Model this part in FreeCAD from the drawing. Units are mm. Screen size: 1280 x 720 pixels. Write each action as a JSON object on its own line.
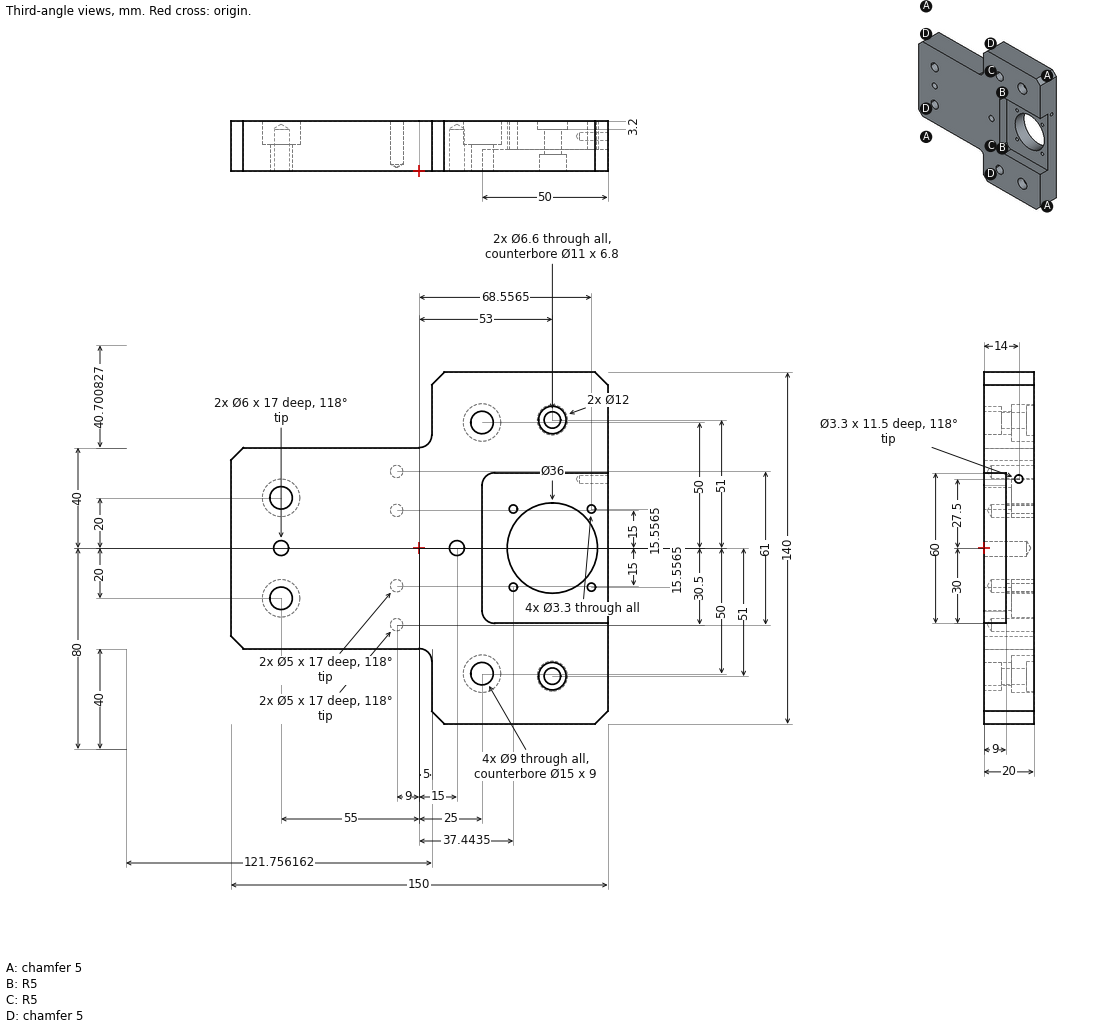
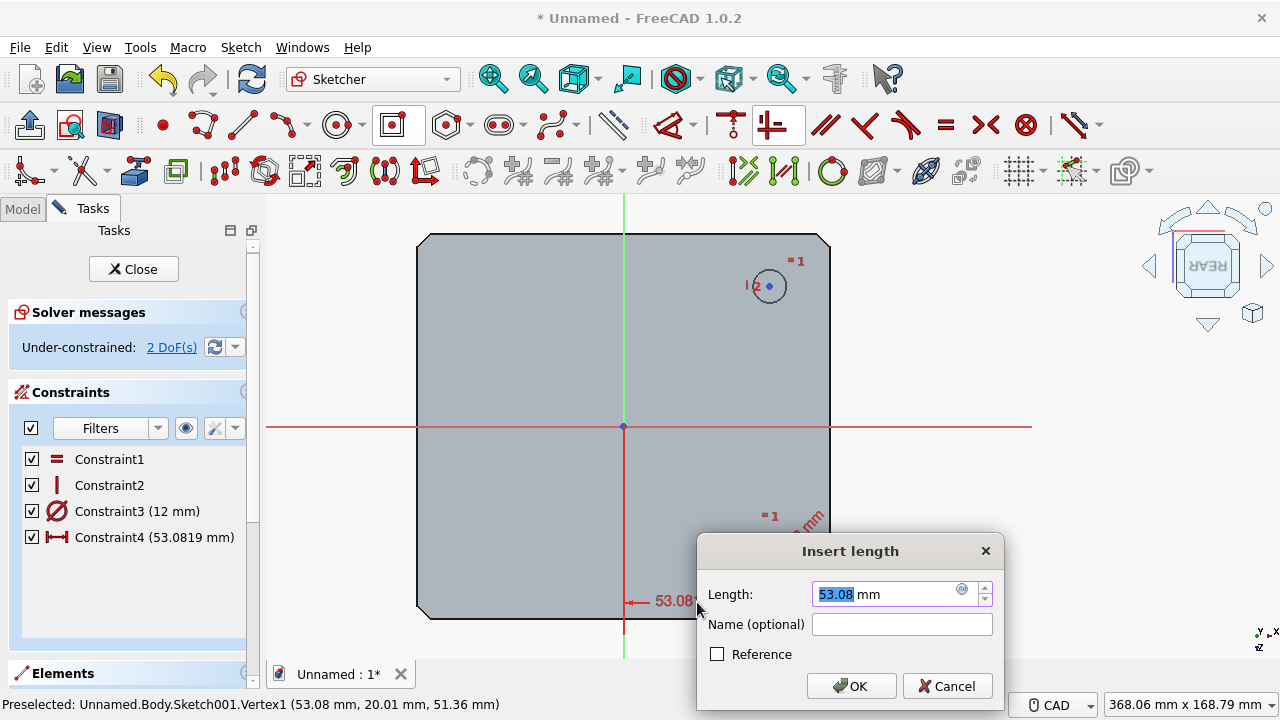
{"action": "type", "text": "53"}
{"action": "key", "text": "Return"}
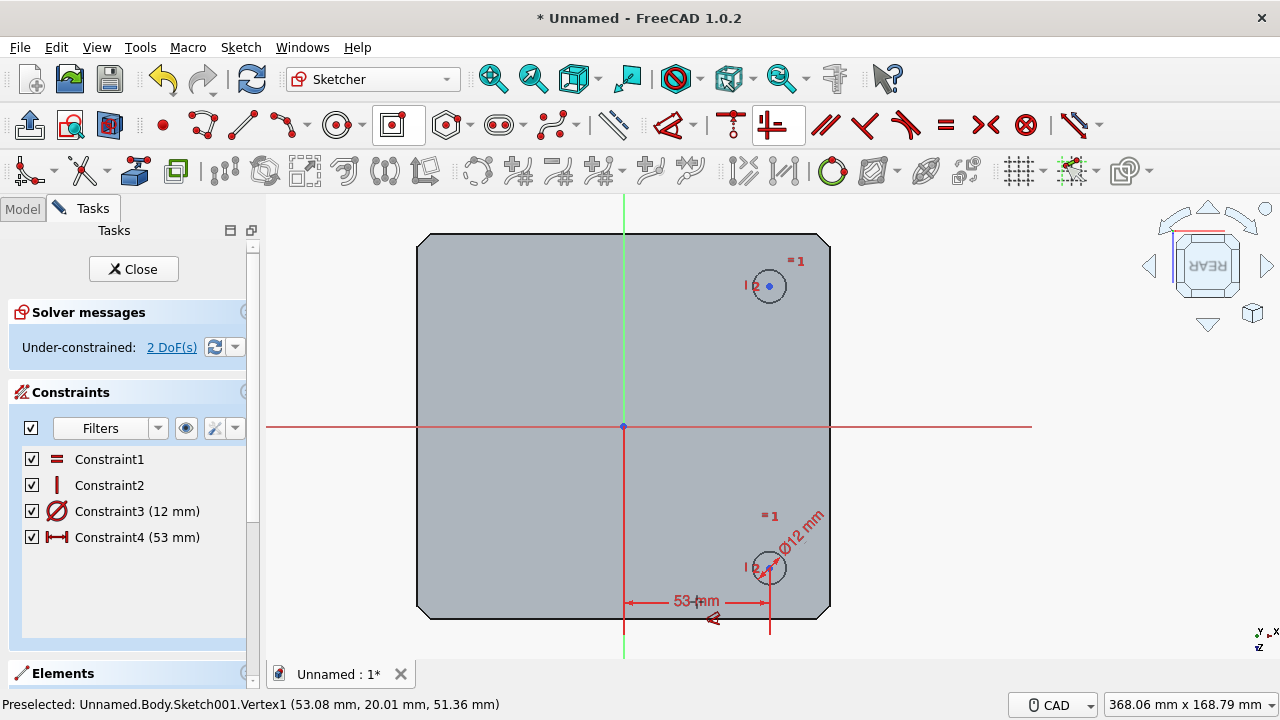
{"action": "left_click", "coordinate": [770, 568]}
{"action": "left_click", "coordinate": [590, 497]}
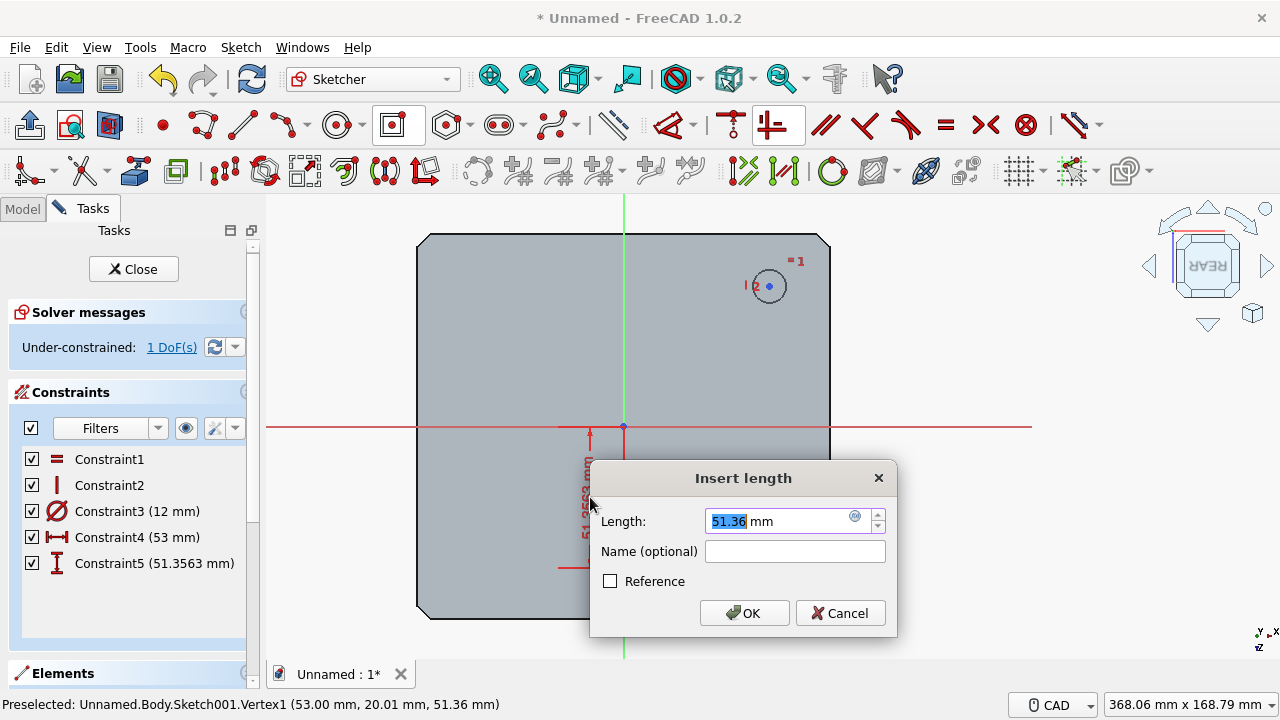
{"action": "type", "text": "51"}
{"action": "key", "text": "Return"}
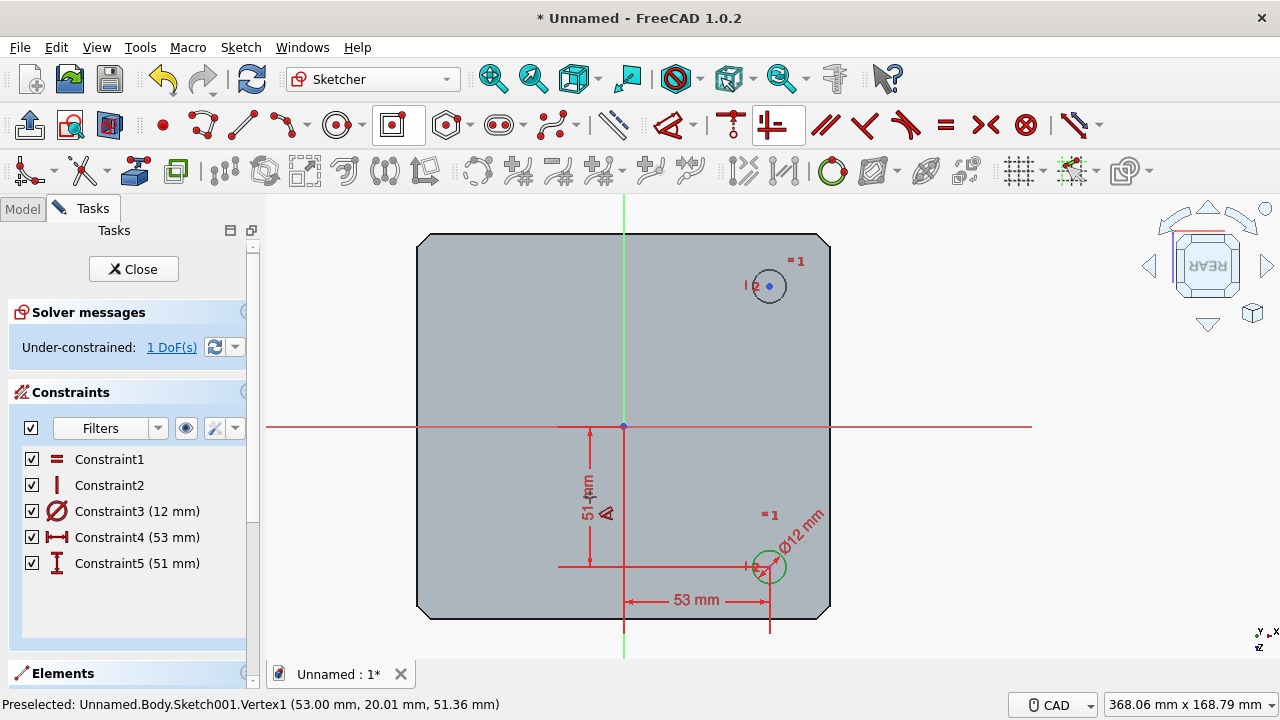
{"action": "left_click", "coordinate": [770, 286]}
{"action": "left_click", "coordinate": [590, 356]}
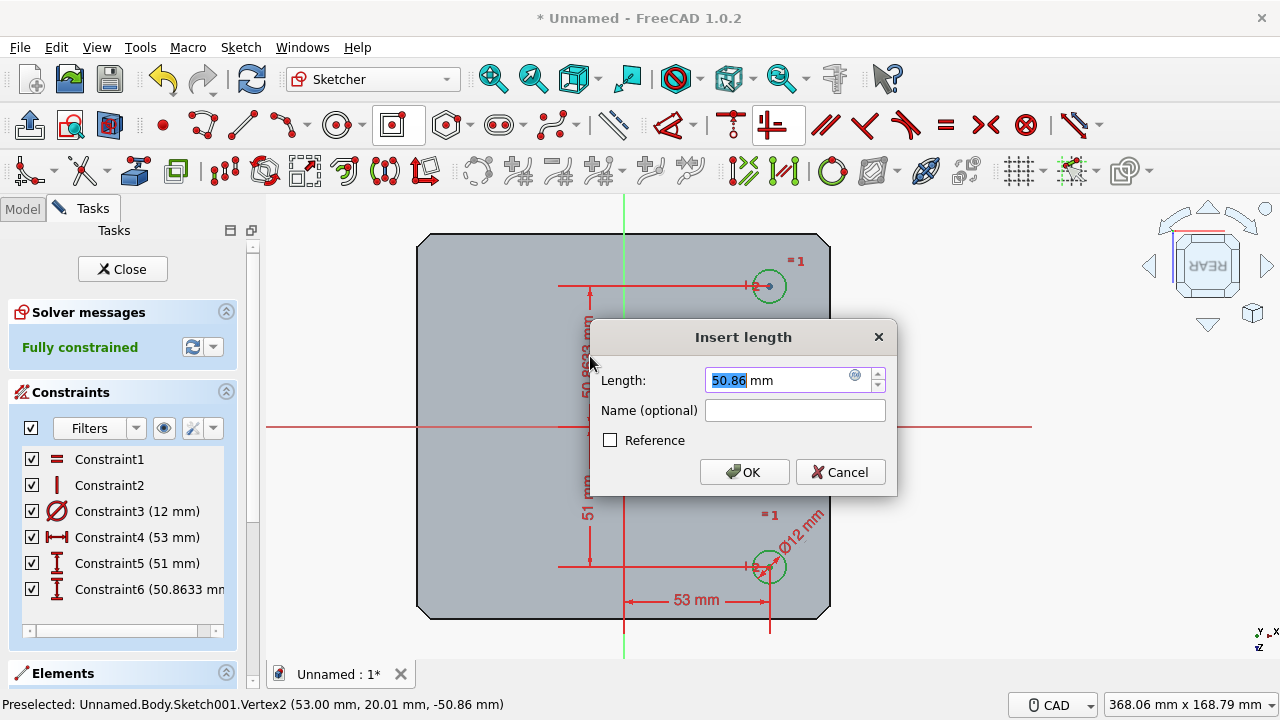
{"action": "type", "text": "51"}
{"action": "key", "text": "Return"}
{"action": "key", "text": "Escape"}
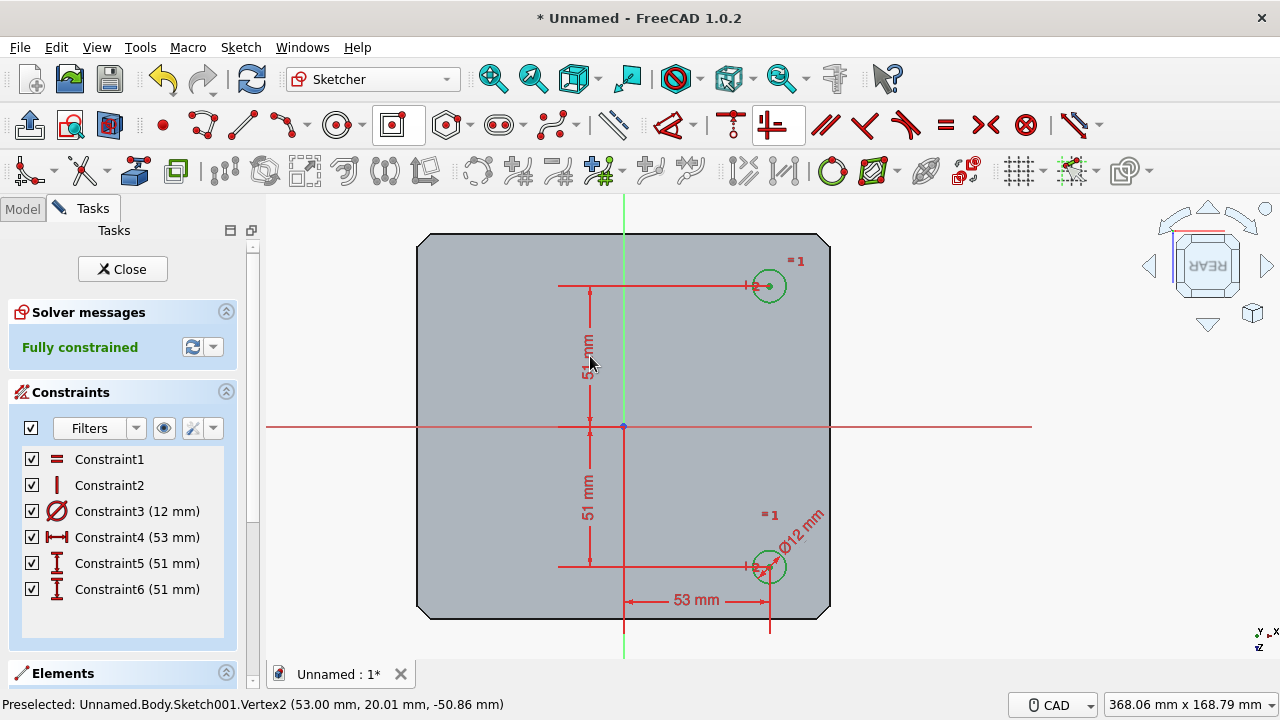
{"action": "left_click", "coordinate": [123, 269]}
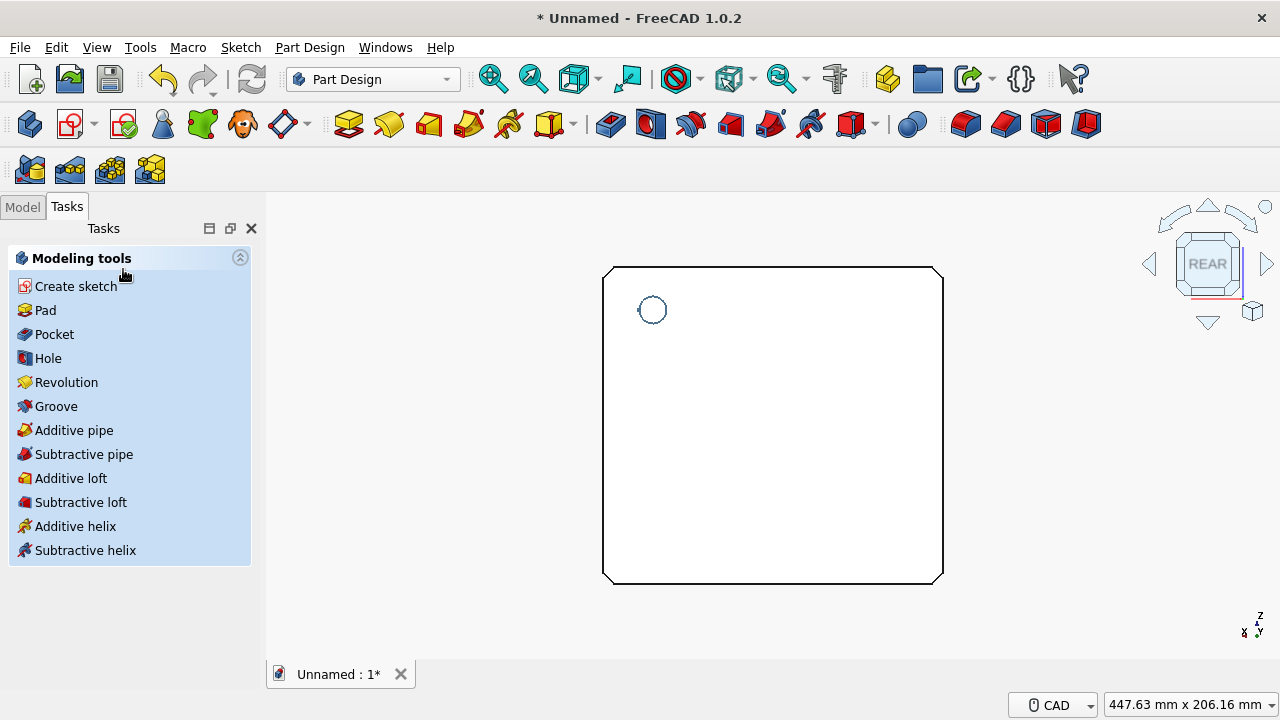
{"action": "left_click", "coordinate": [612, 124]}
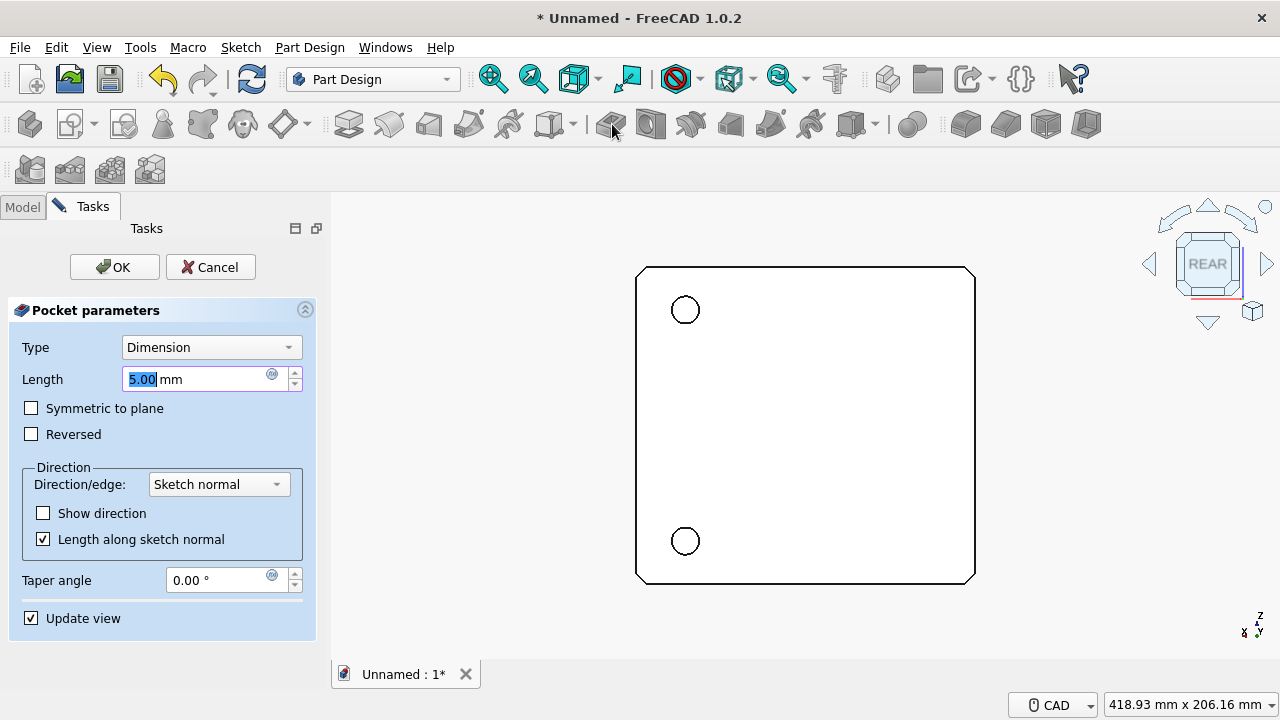
{"action": "type", "text": "3.2"}
{"action": "key", "text": "Tab"}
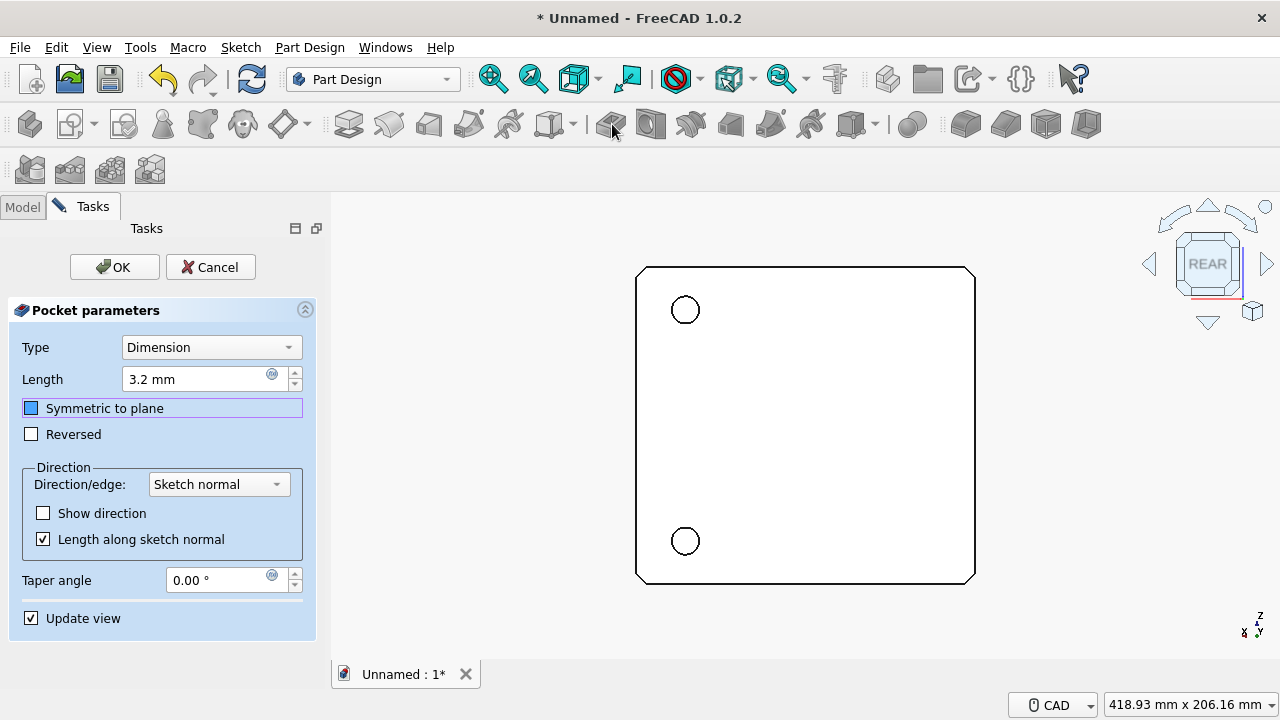
{"action": "left_click", "coordinate": [115, 267]}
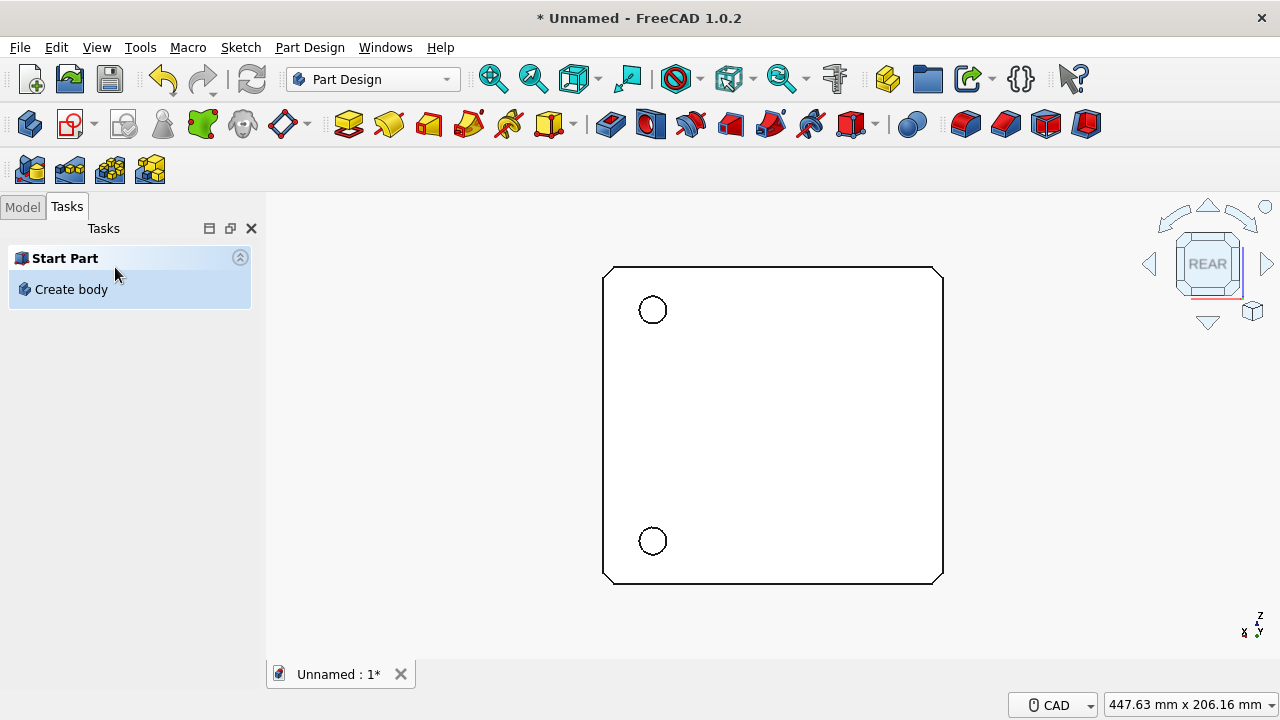
{"action": "left_click", "coordinate": [773, 424]}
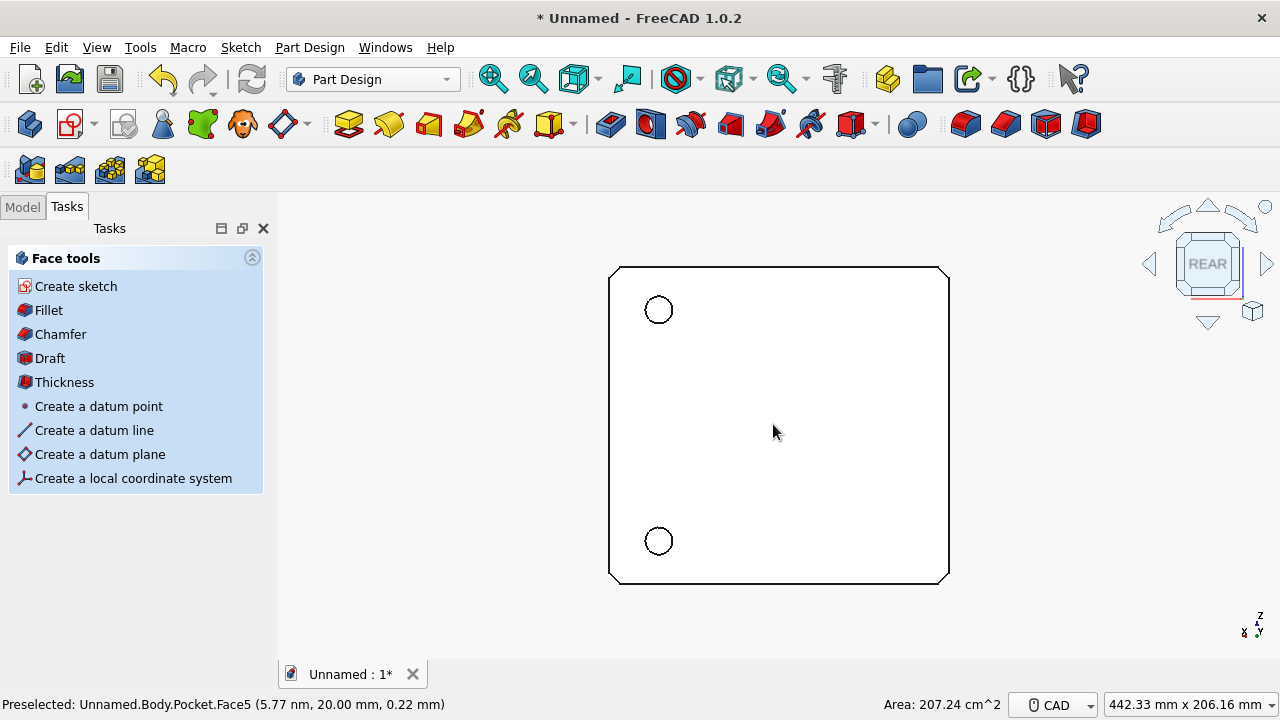
{"action": "left_click", "coordinate": [70, 124]}